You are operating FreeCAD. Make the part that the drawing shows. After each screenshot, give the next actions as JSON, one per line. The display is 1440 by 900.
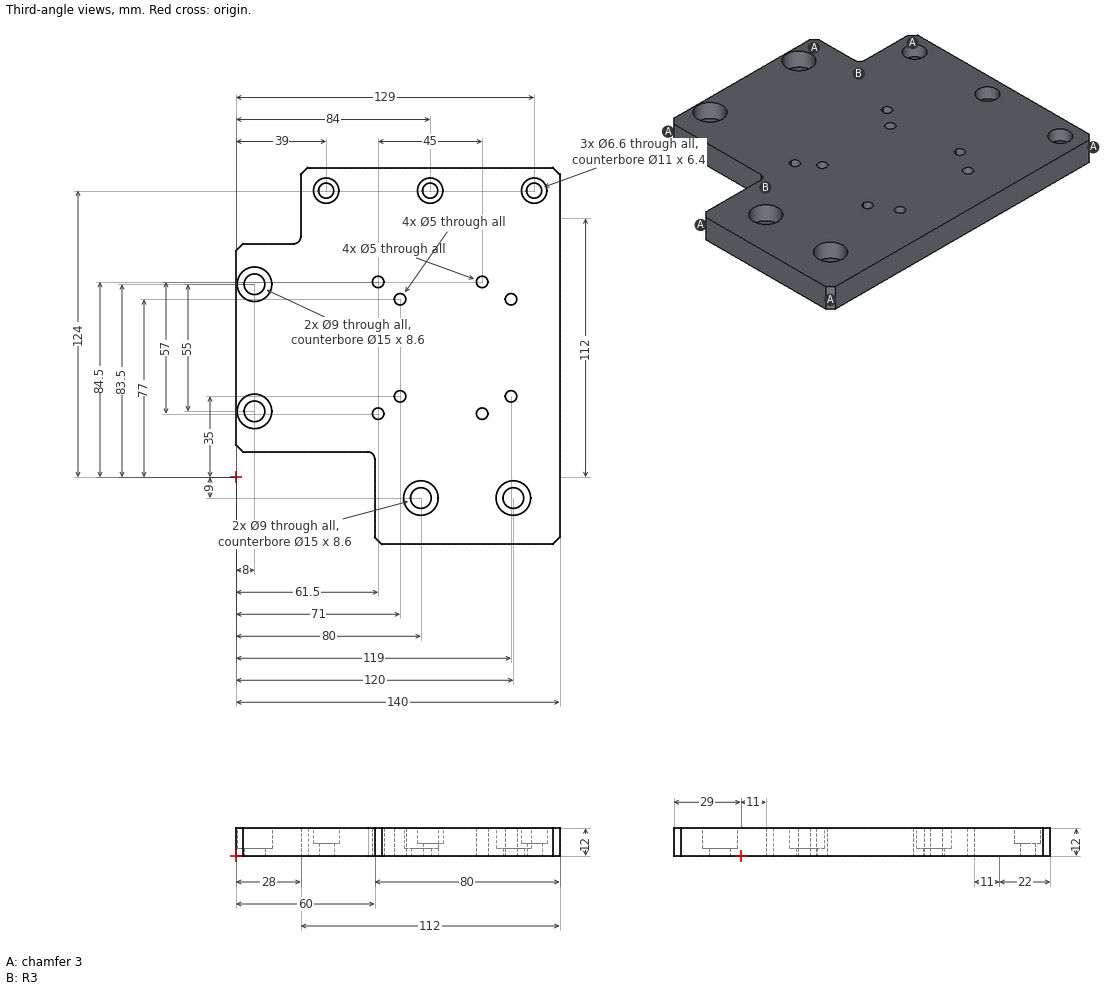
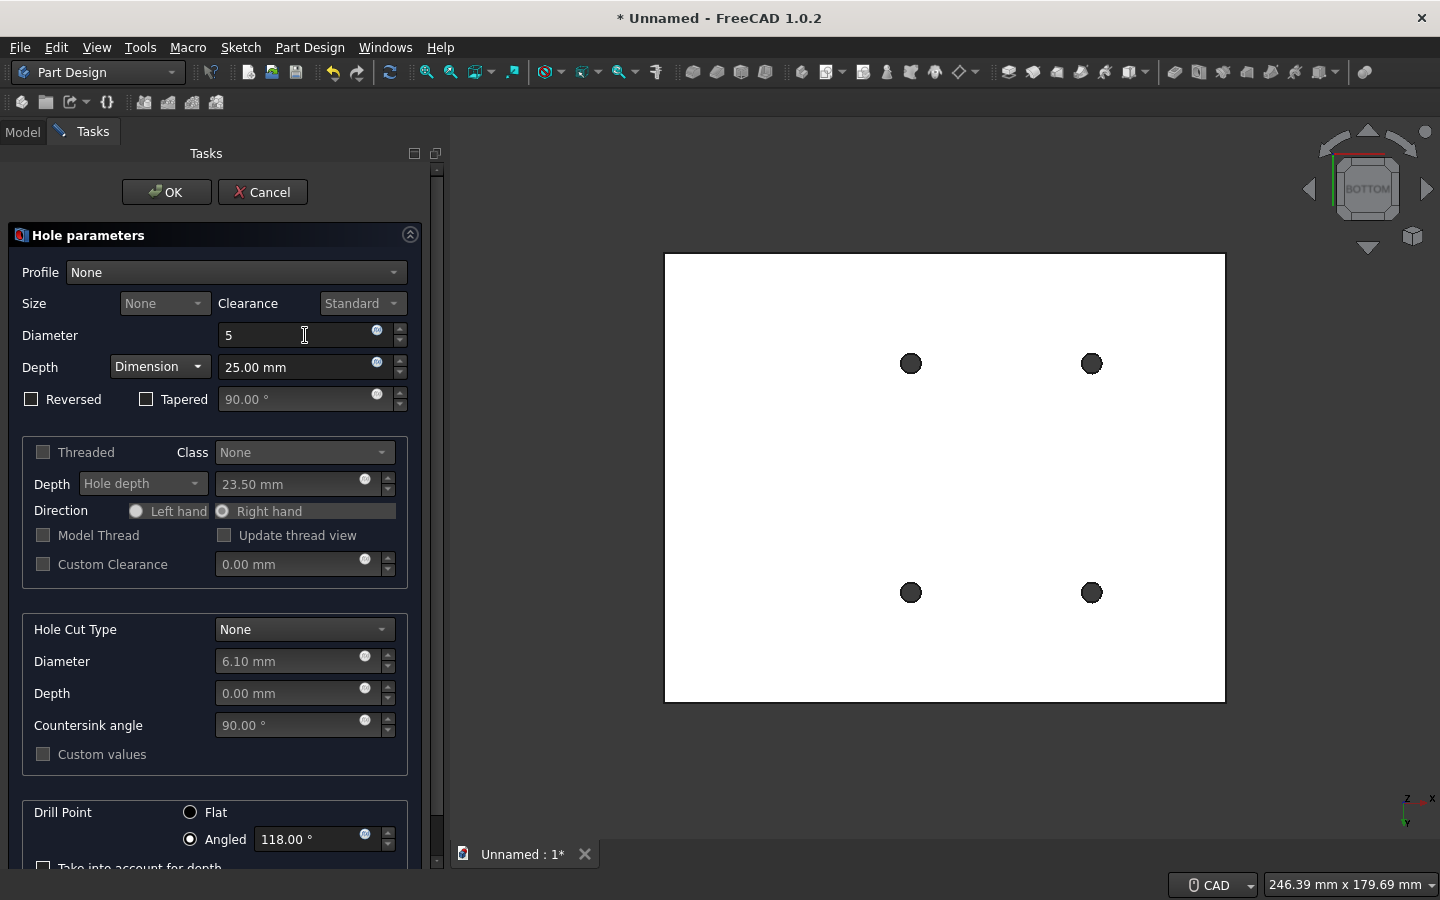
{"action": "left_click", "coordinate": [161, 366]}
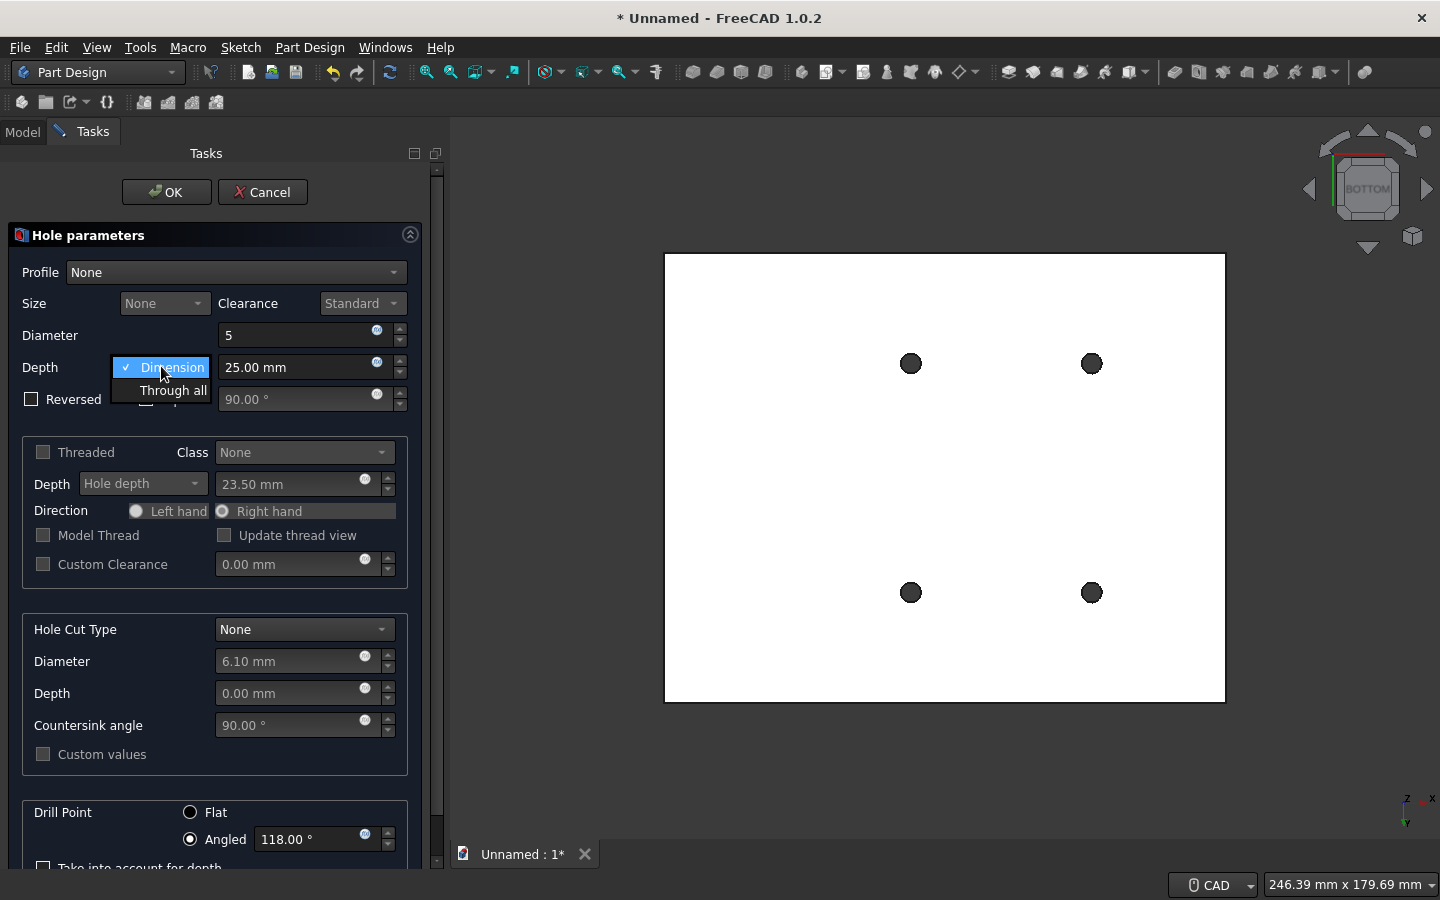
{"action": "left_click", "coordinate": [160, 390]}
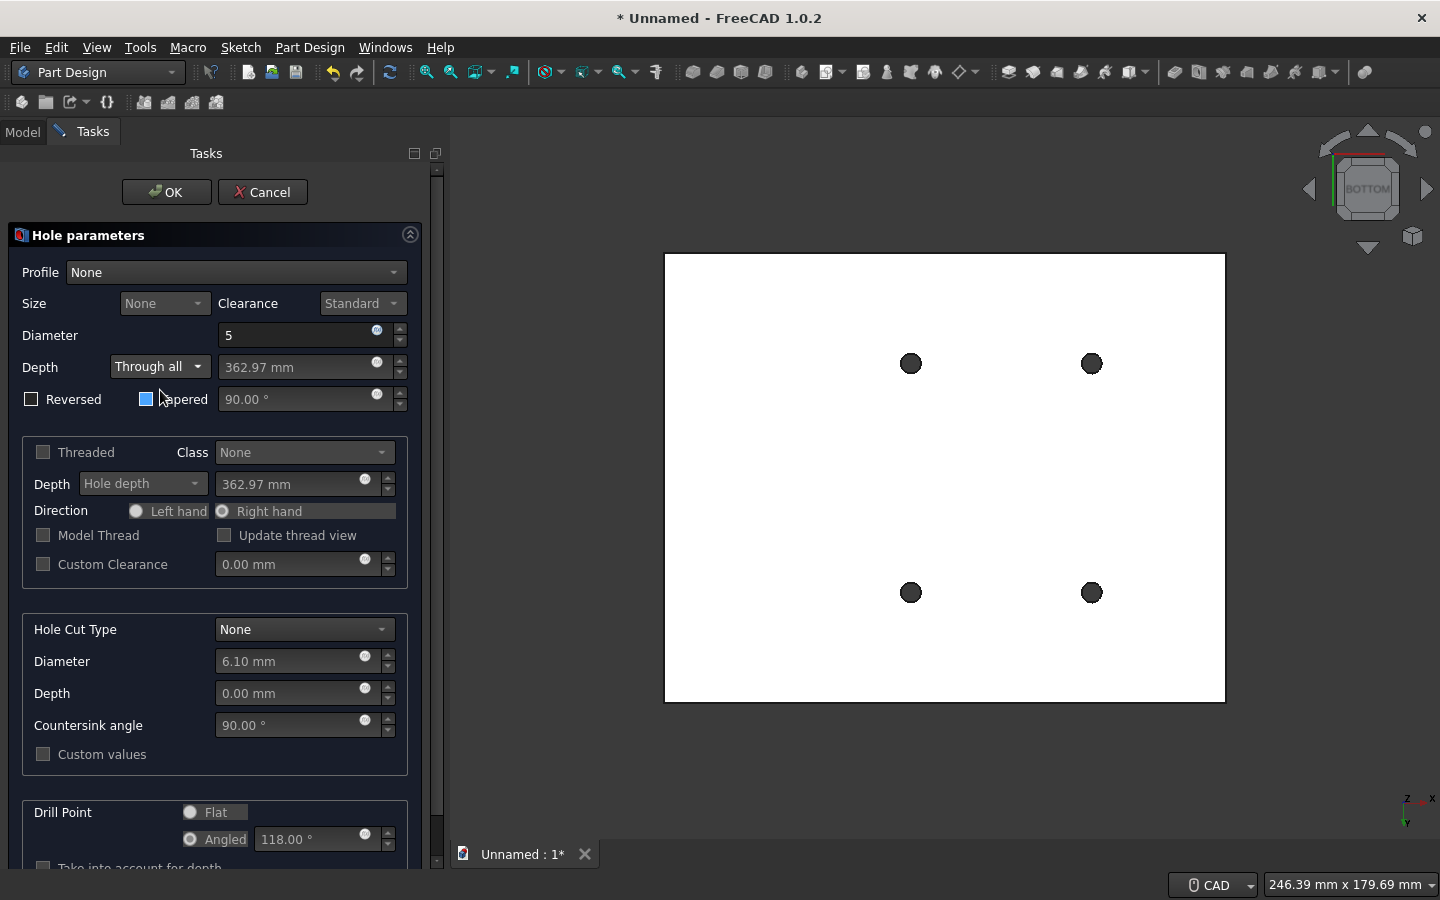
{"action": "left_click", "coordinate": [167, 192]}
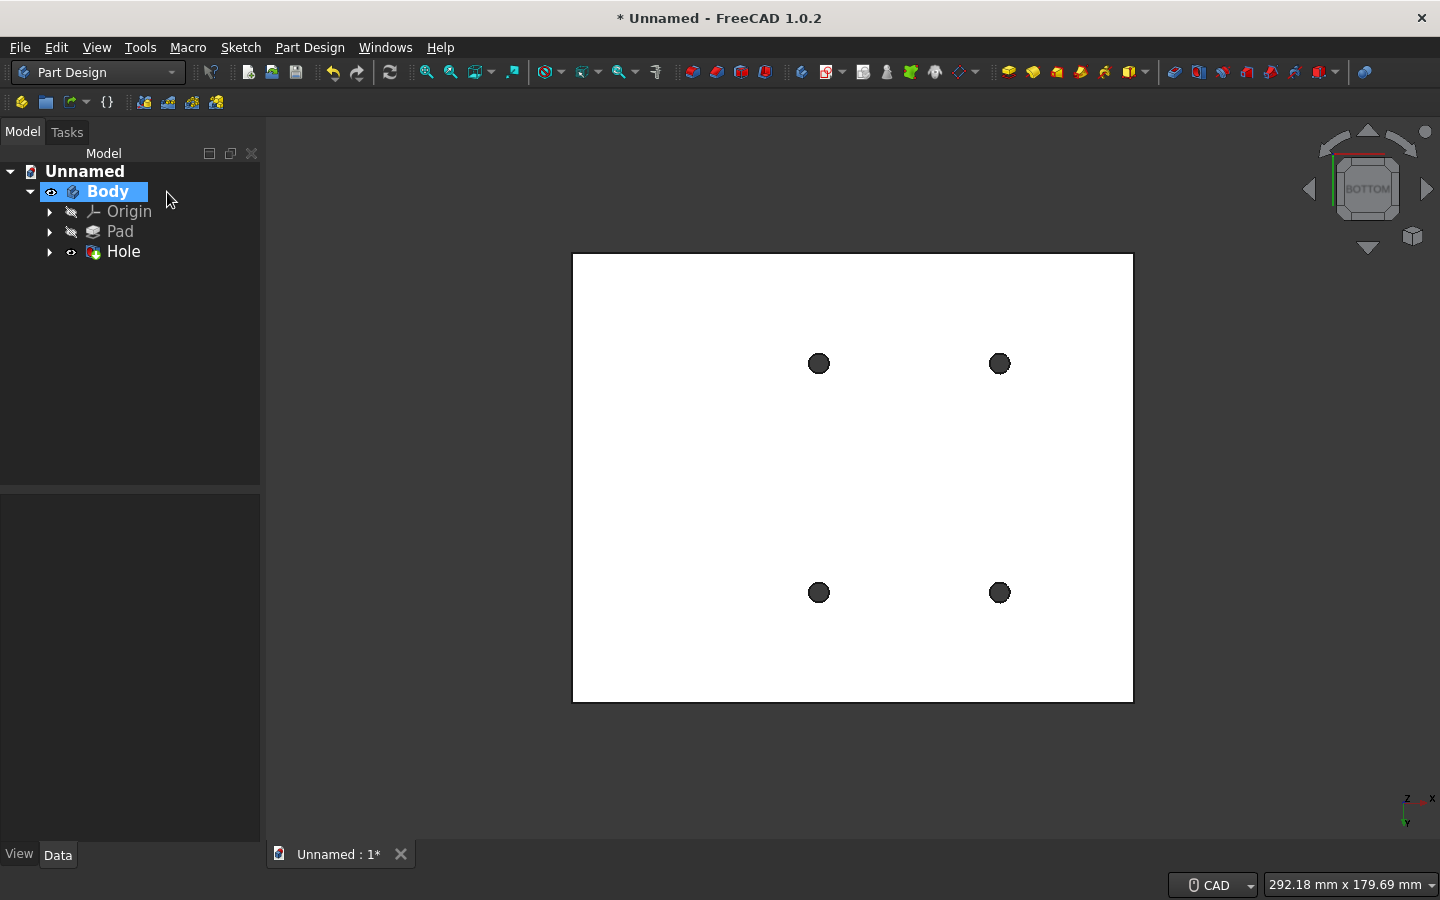
{"action": "key", "text": "0"}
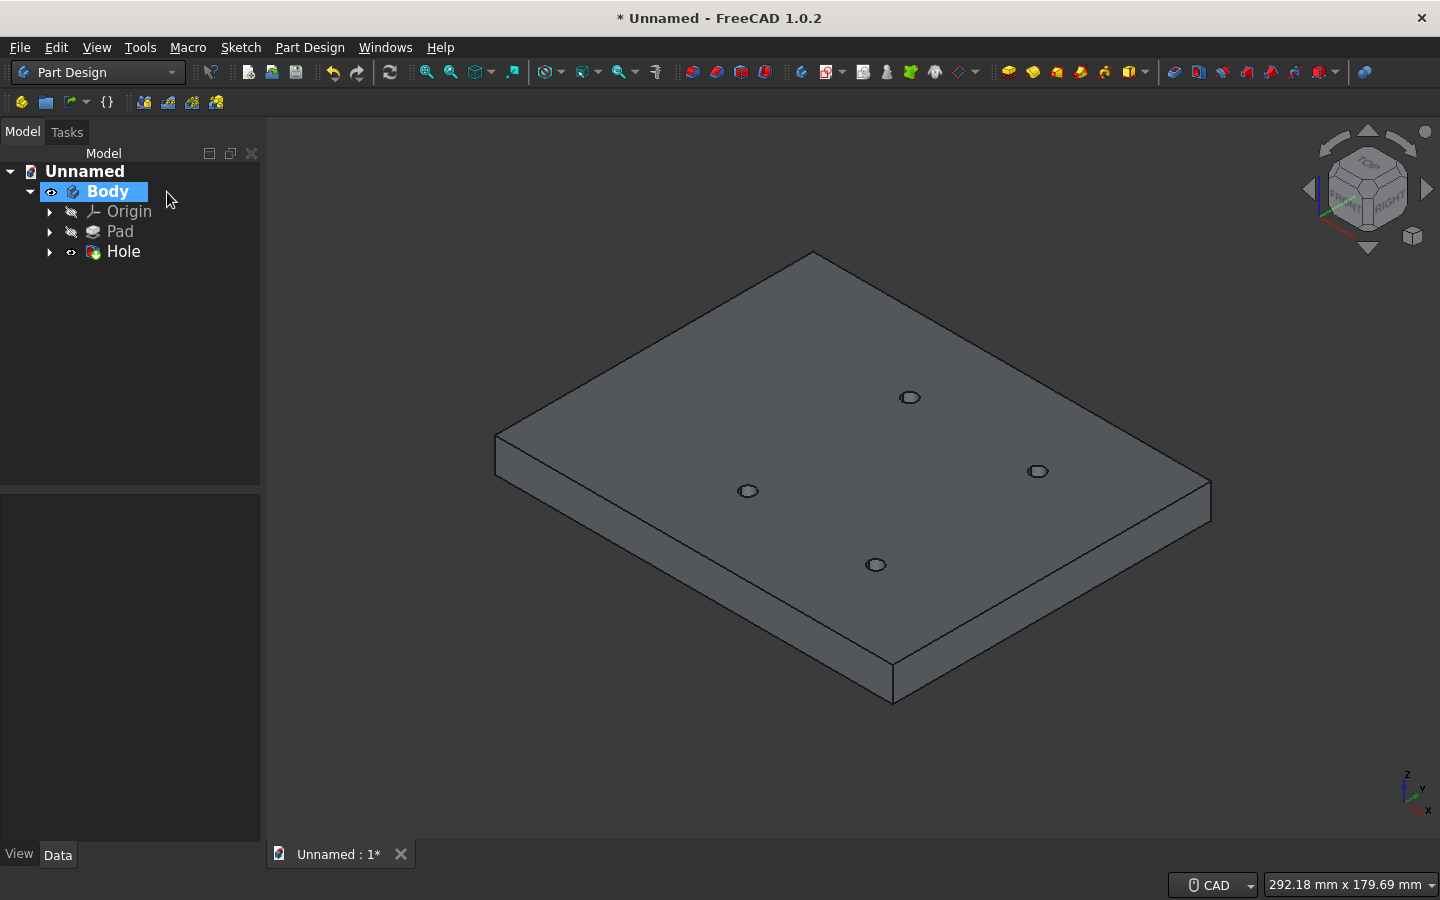
{"action": "left_click", "coordinate": [910, 490]}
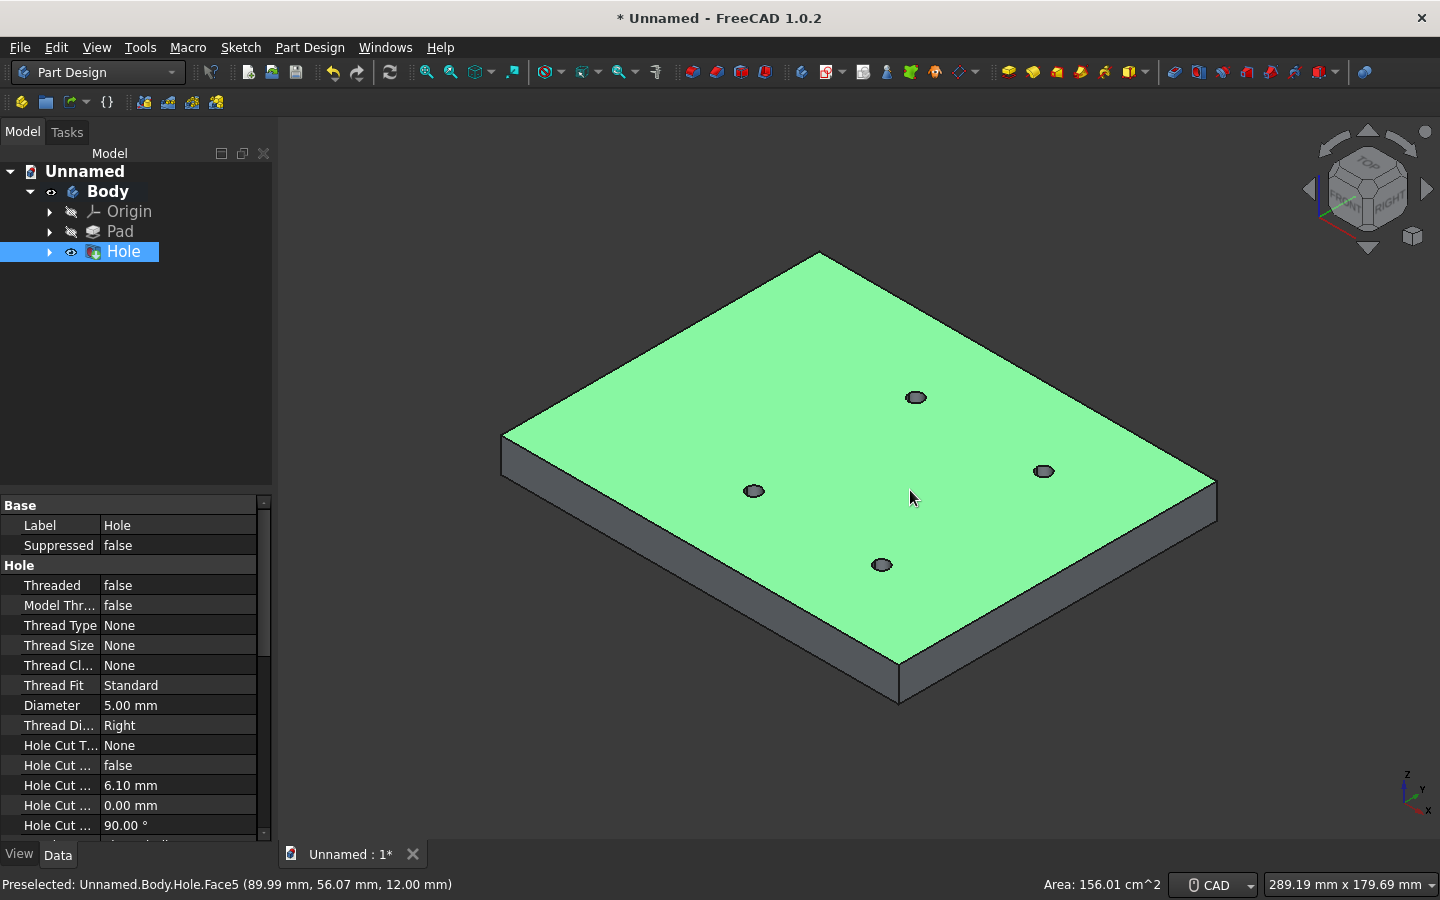
{"action": "left_click", "coordinate": [826, 72]}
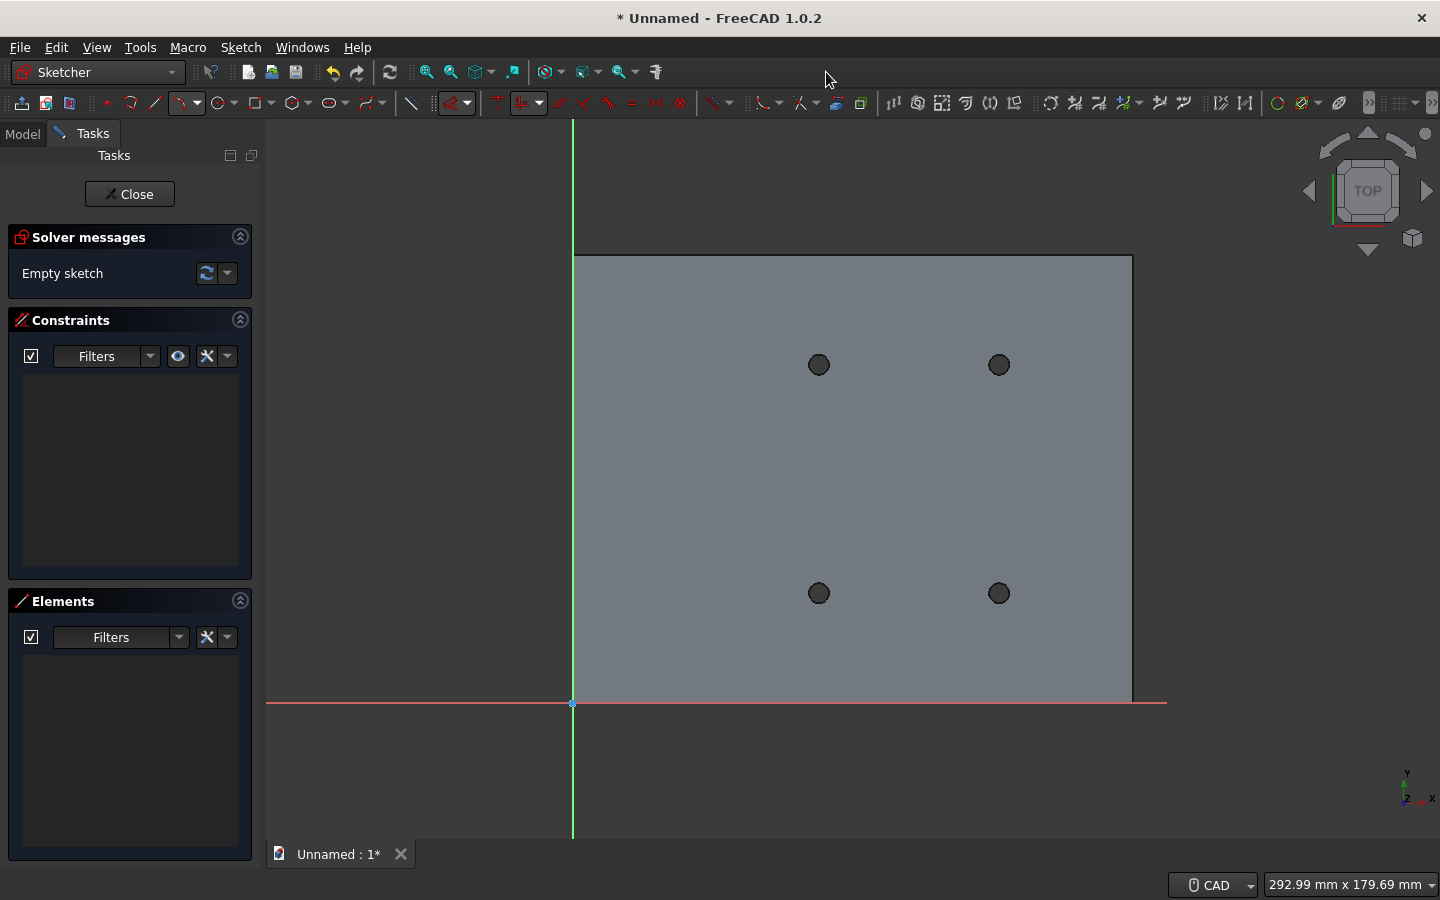
{"action": "scroll", "coordinate": [880, 677], "scroll_direction": "up", "scroll_amount": 2}